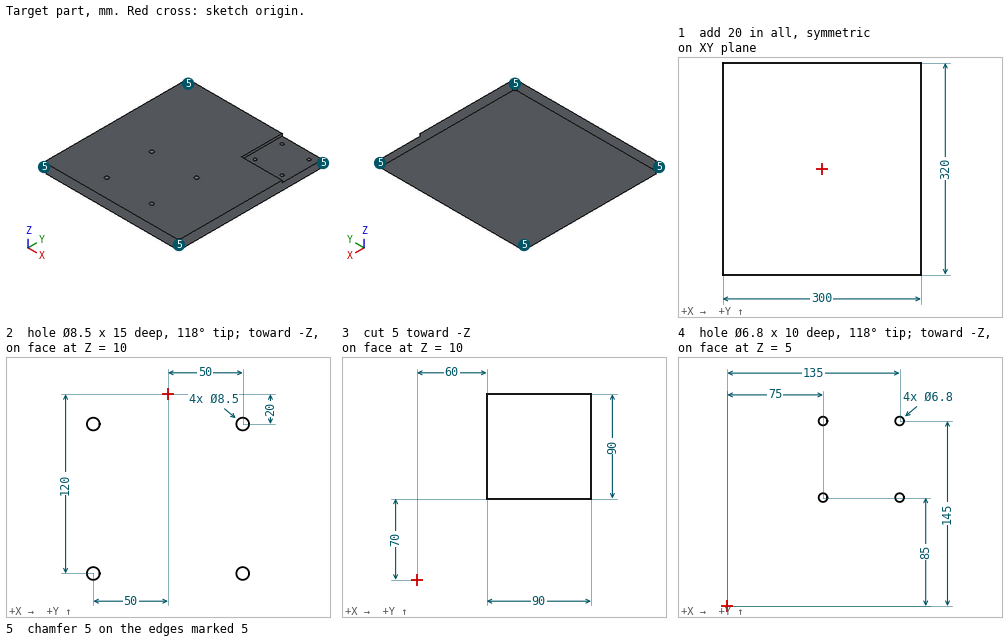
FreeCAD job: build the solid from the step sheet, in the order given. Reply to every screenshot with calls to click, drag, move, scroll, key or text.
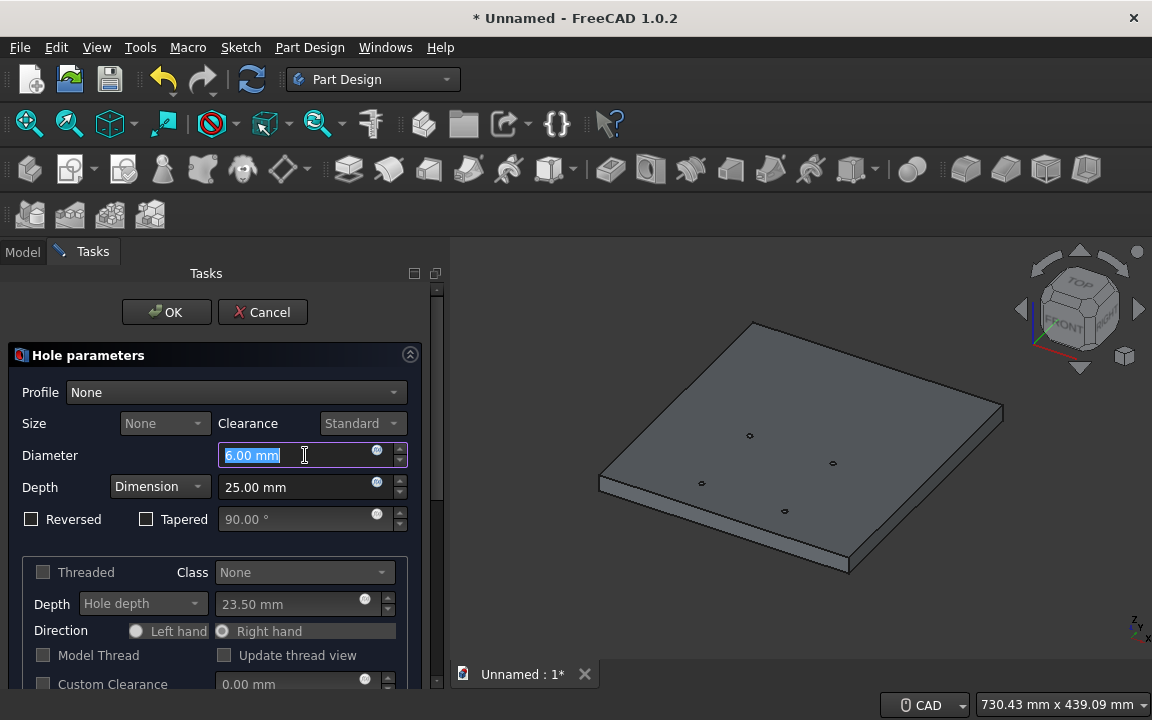
text(8.5)
key(Tab)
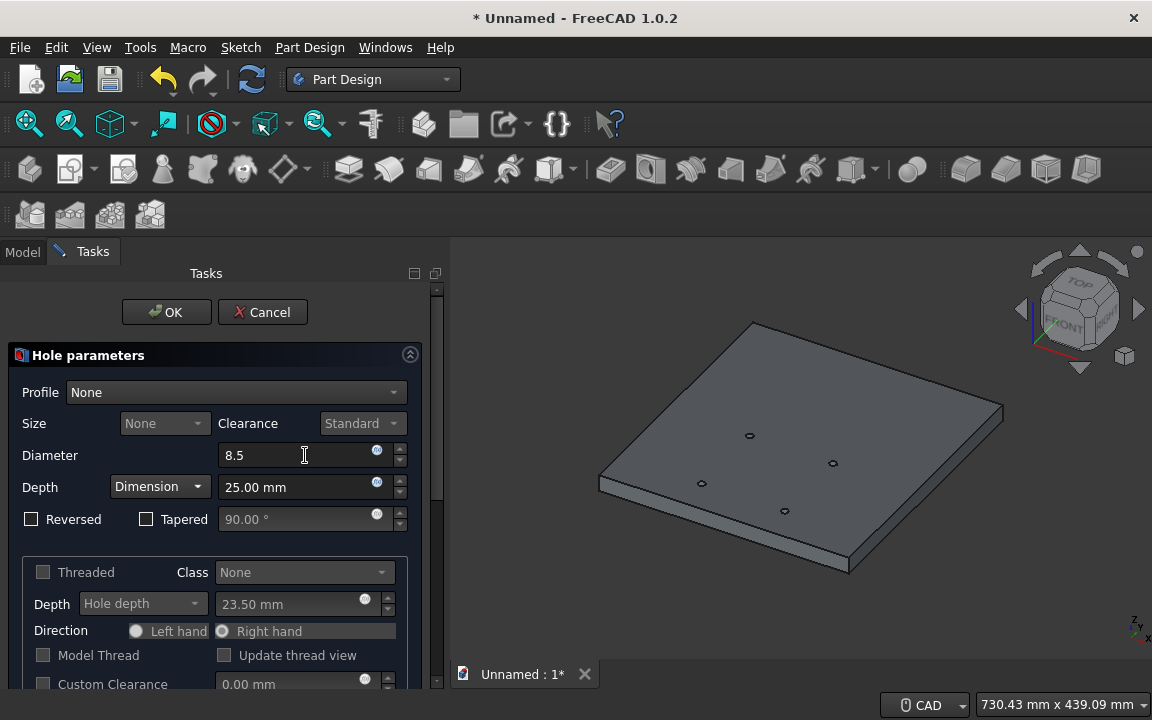
triple_click(305, 487)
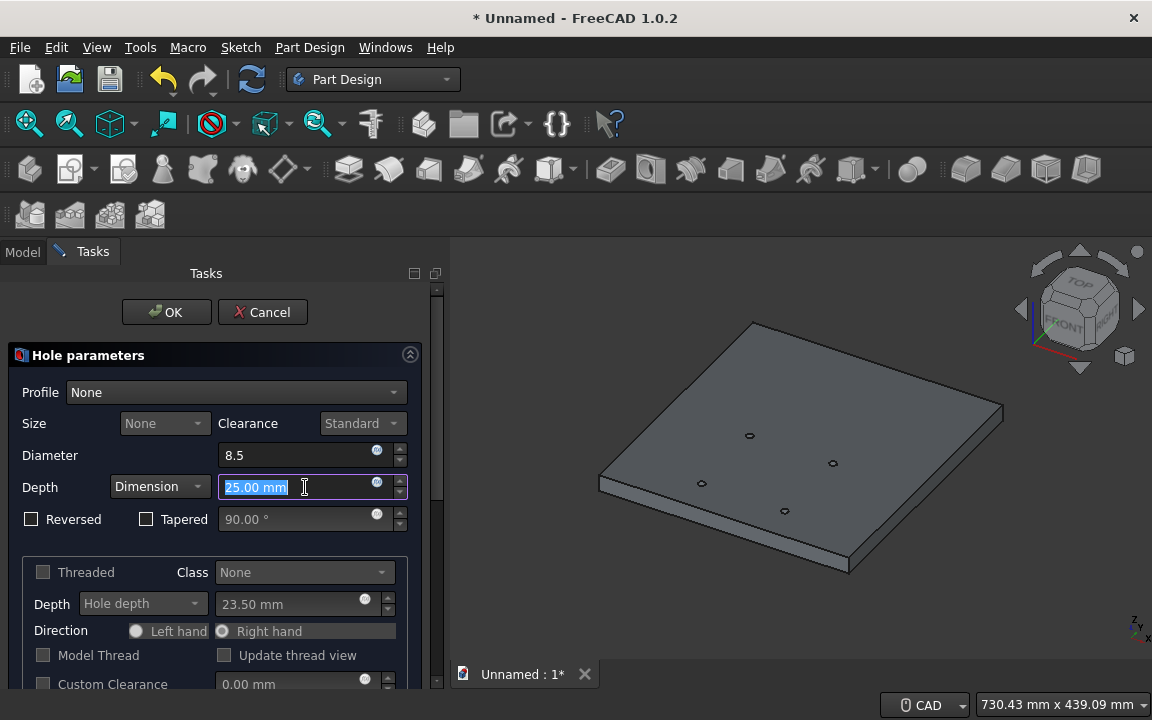
text(15)
key(Tab)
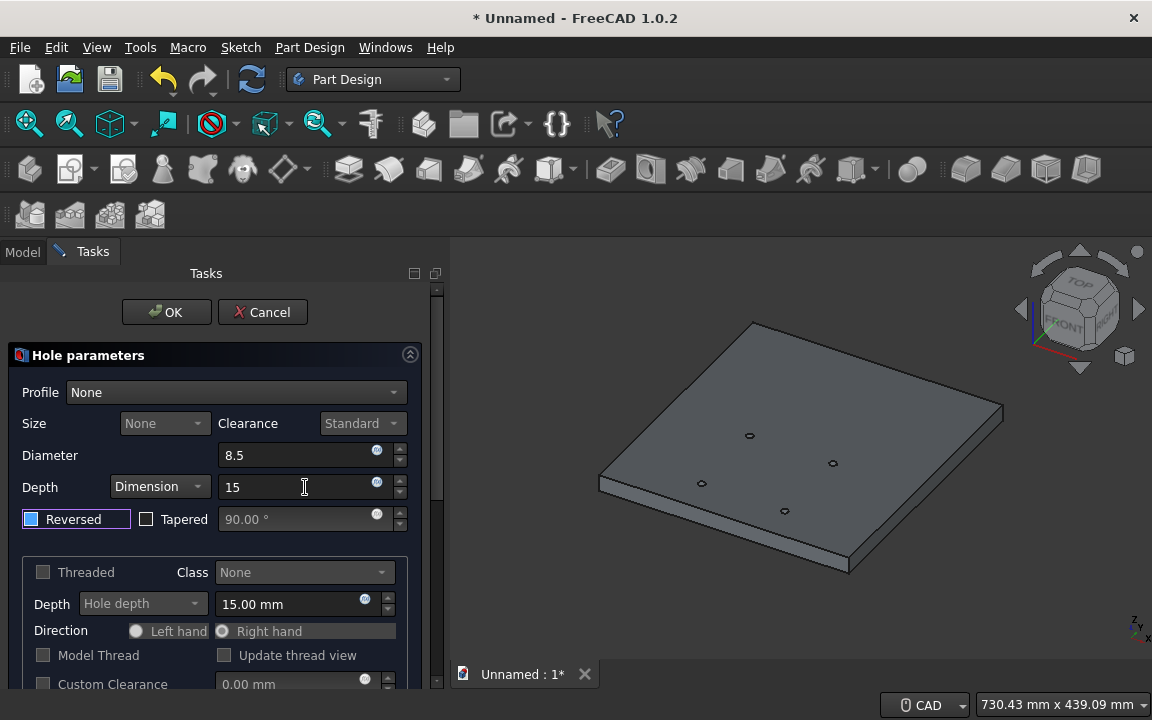
click(167, 312)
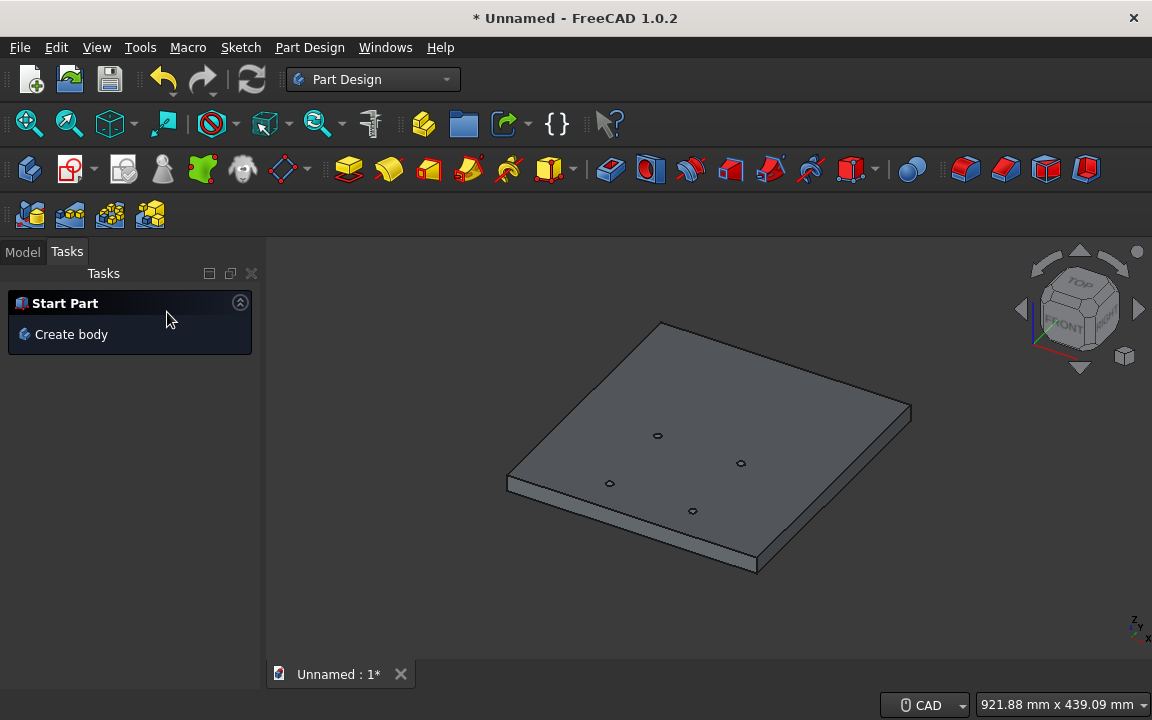
click(731, 417)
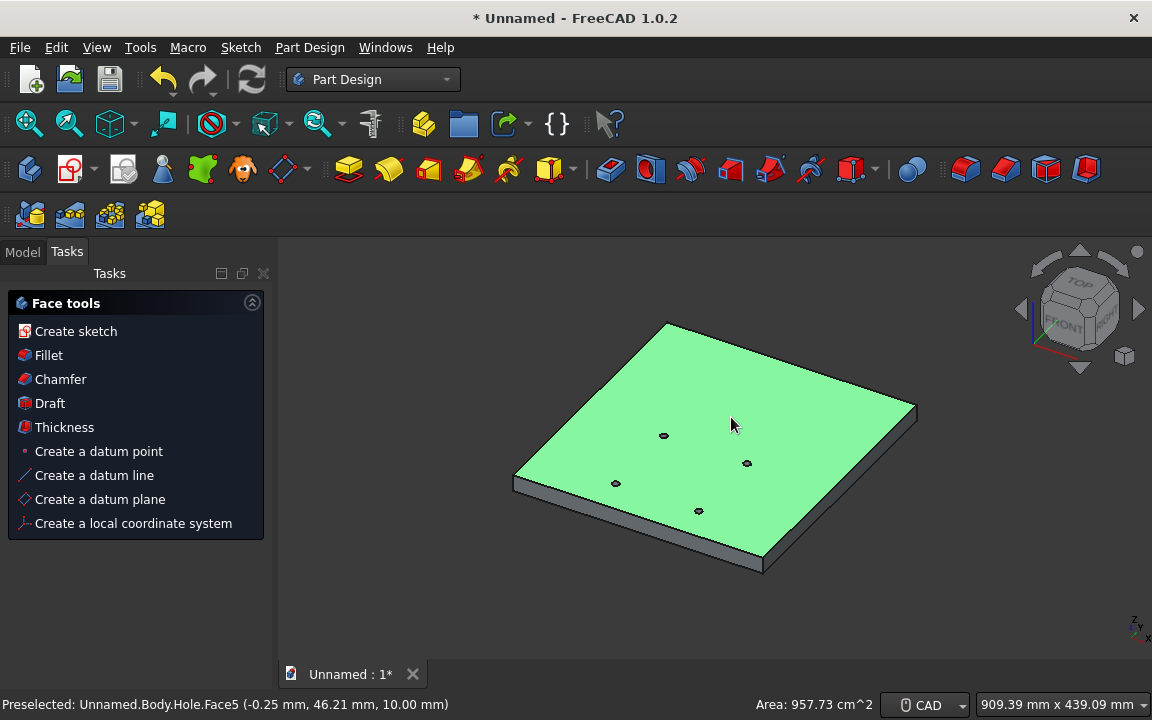
click(70, 170)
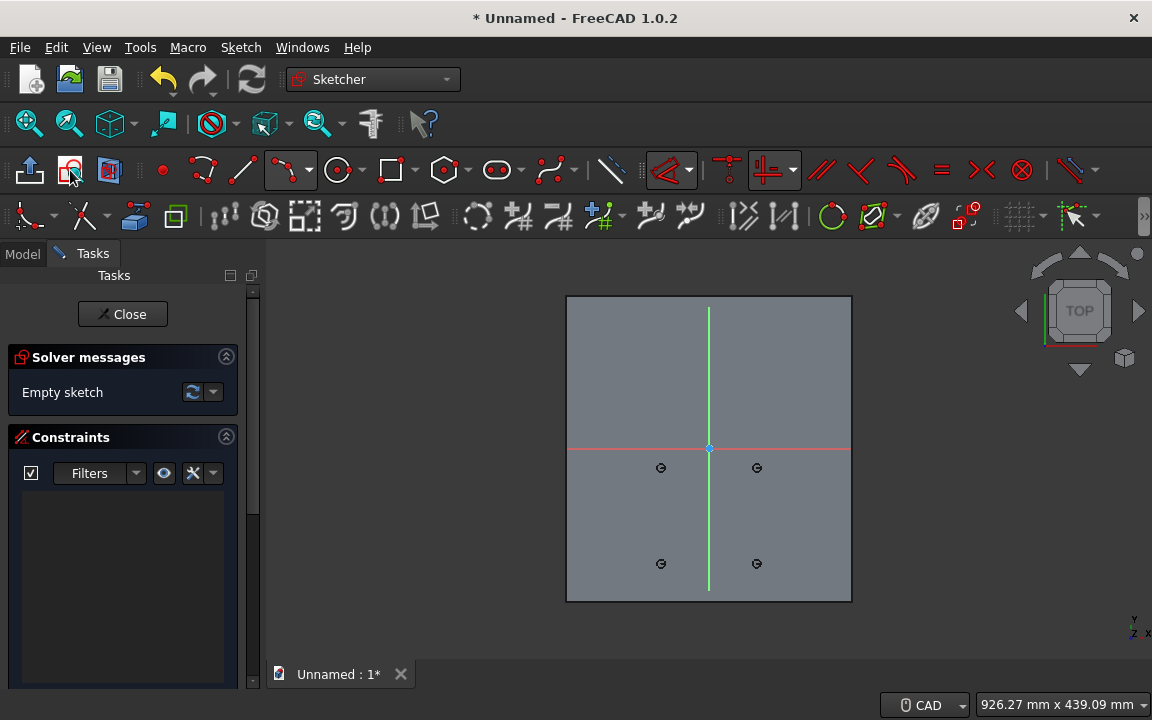
scroll(951, 279, up, 3)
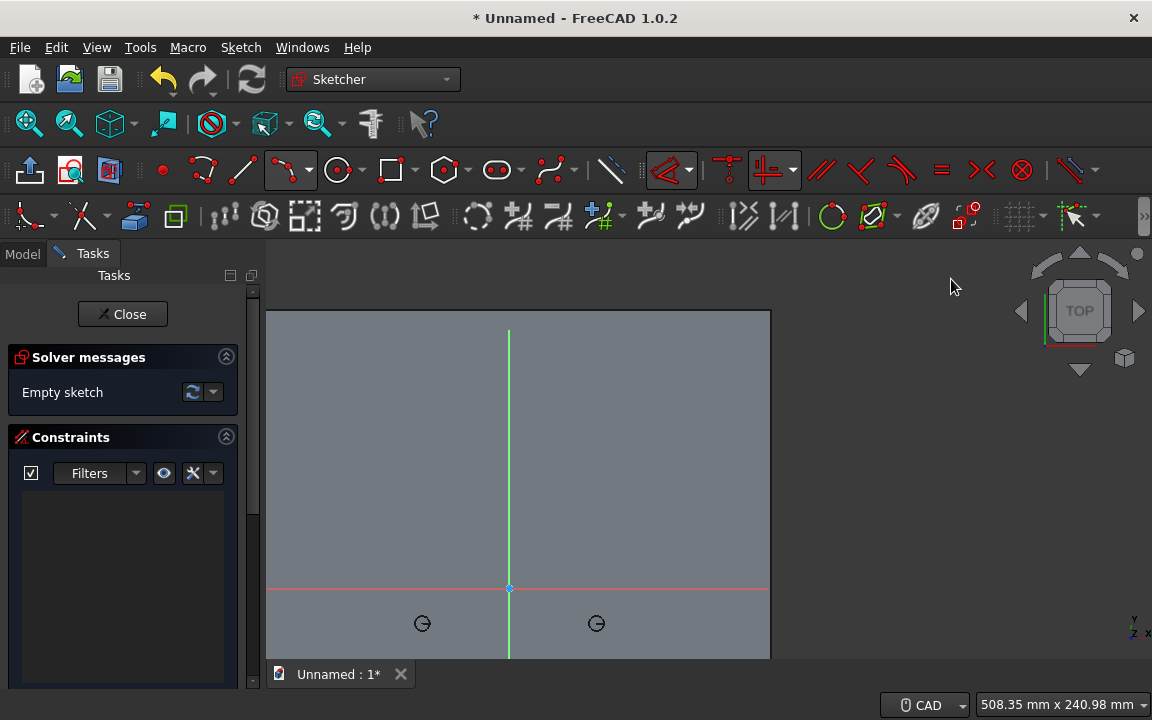
key(g)
key(r)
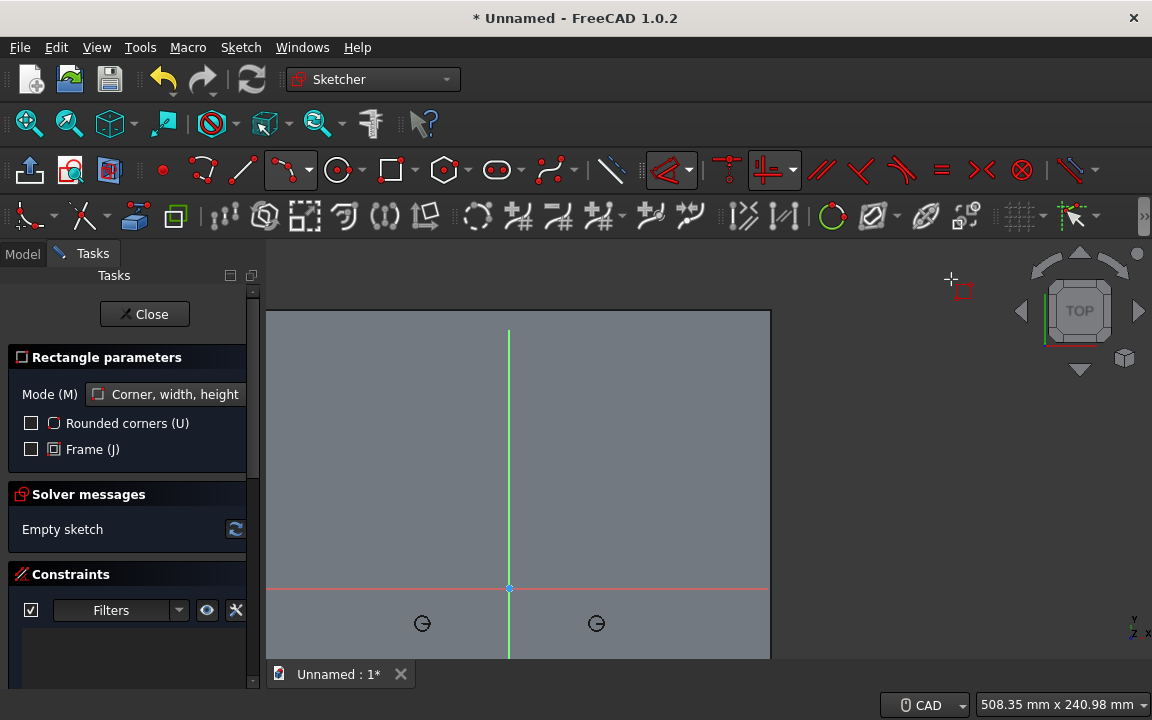
click(614, 310)
move(771, 467)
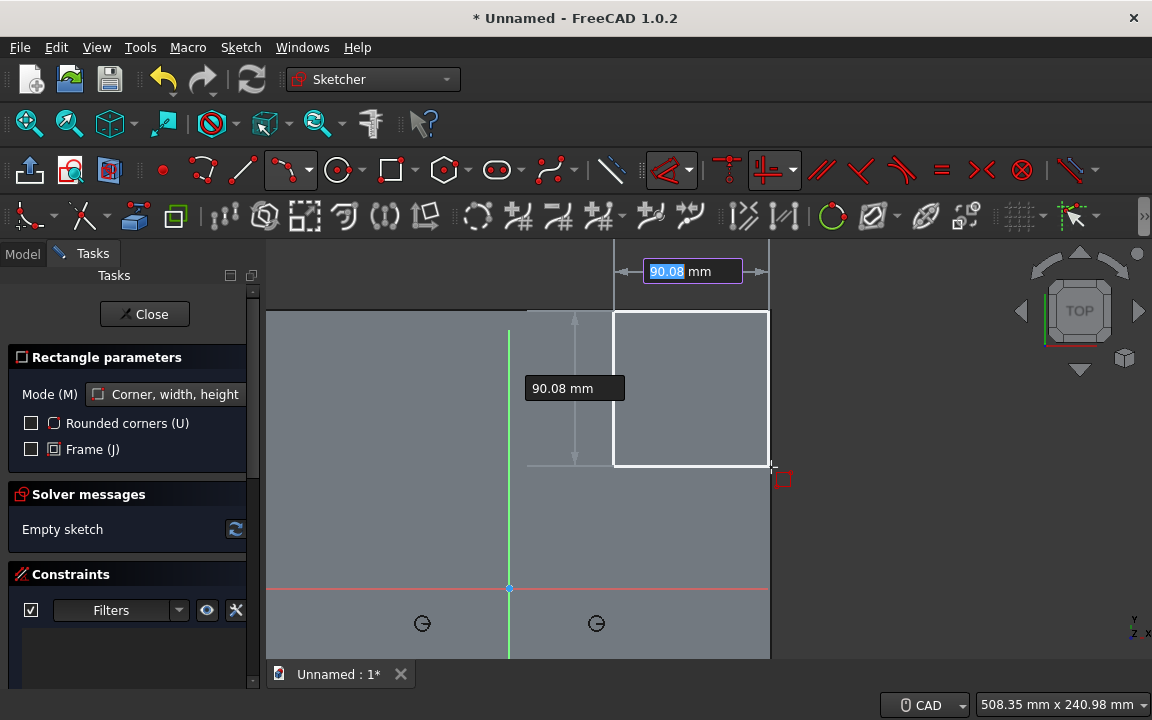
text(90)
key(Tab)
text(90)
key(Return)
key(Escape)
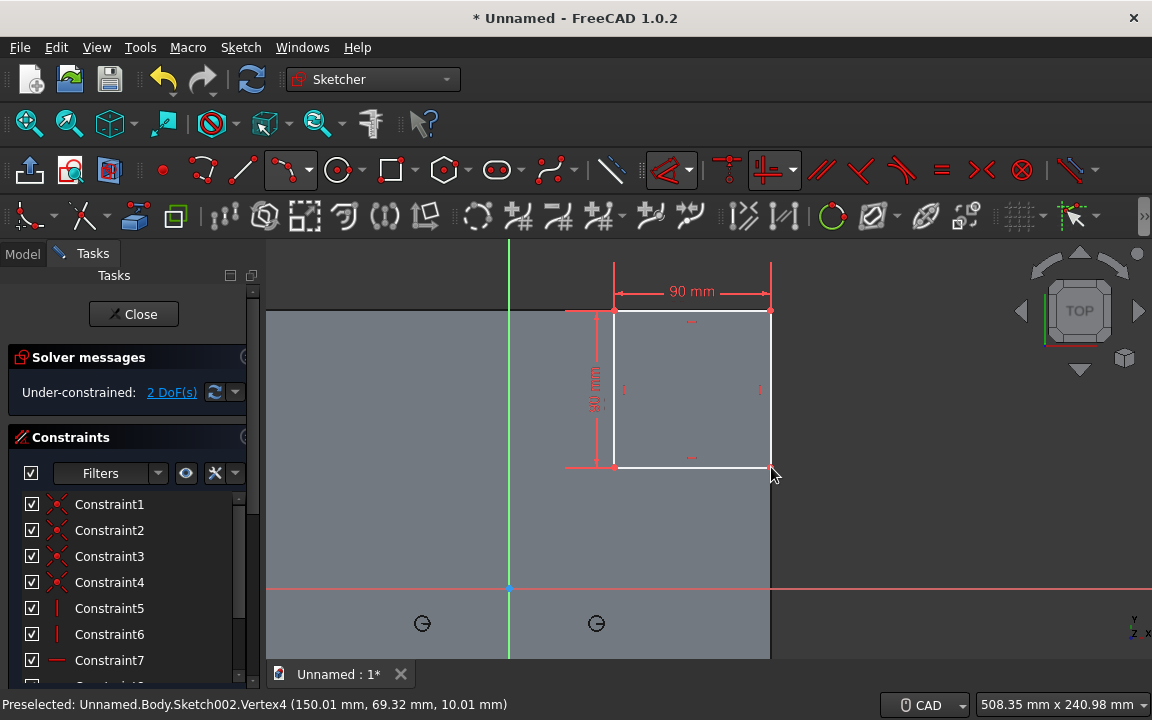
click(614, 311)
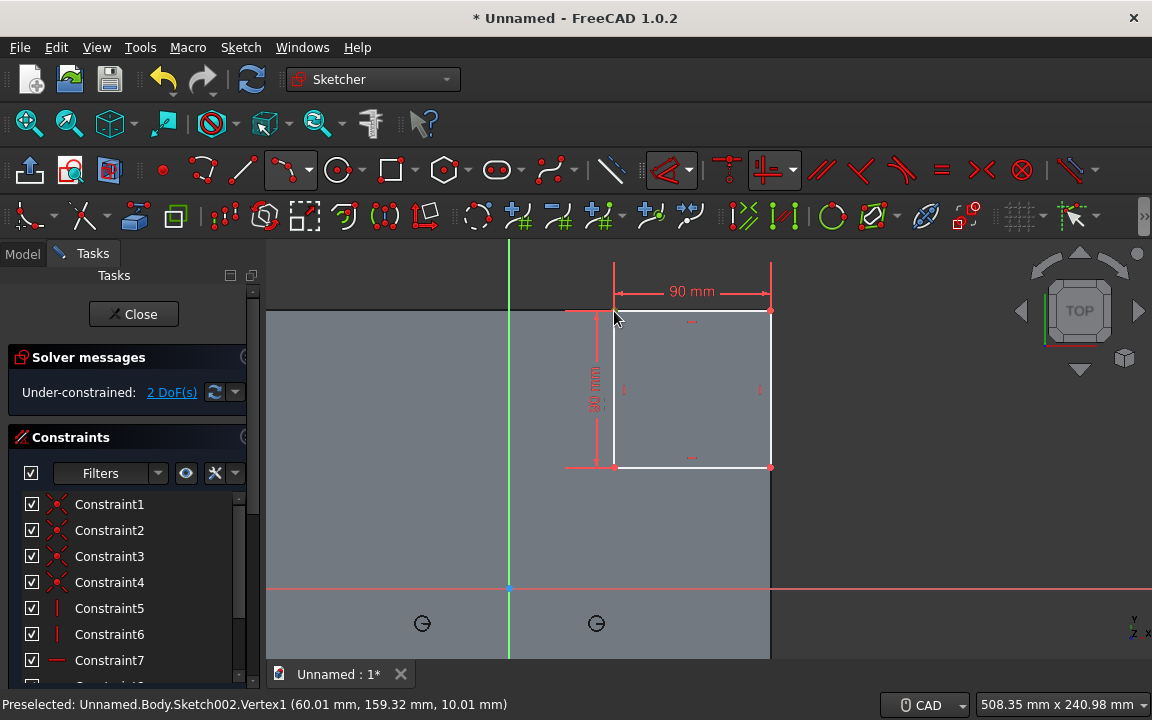
key(l)